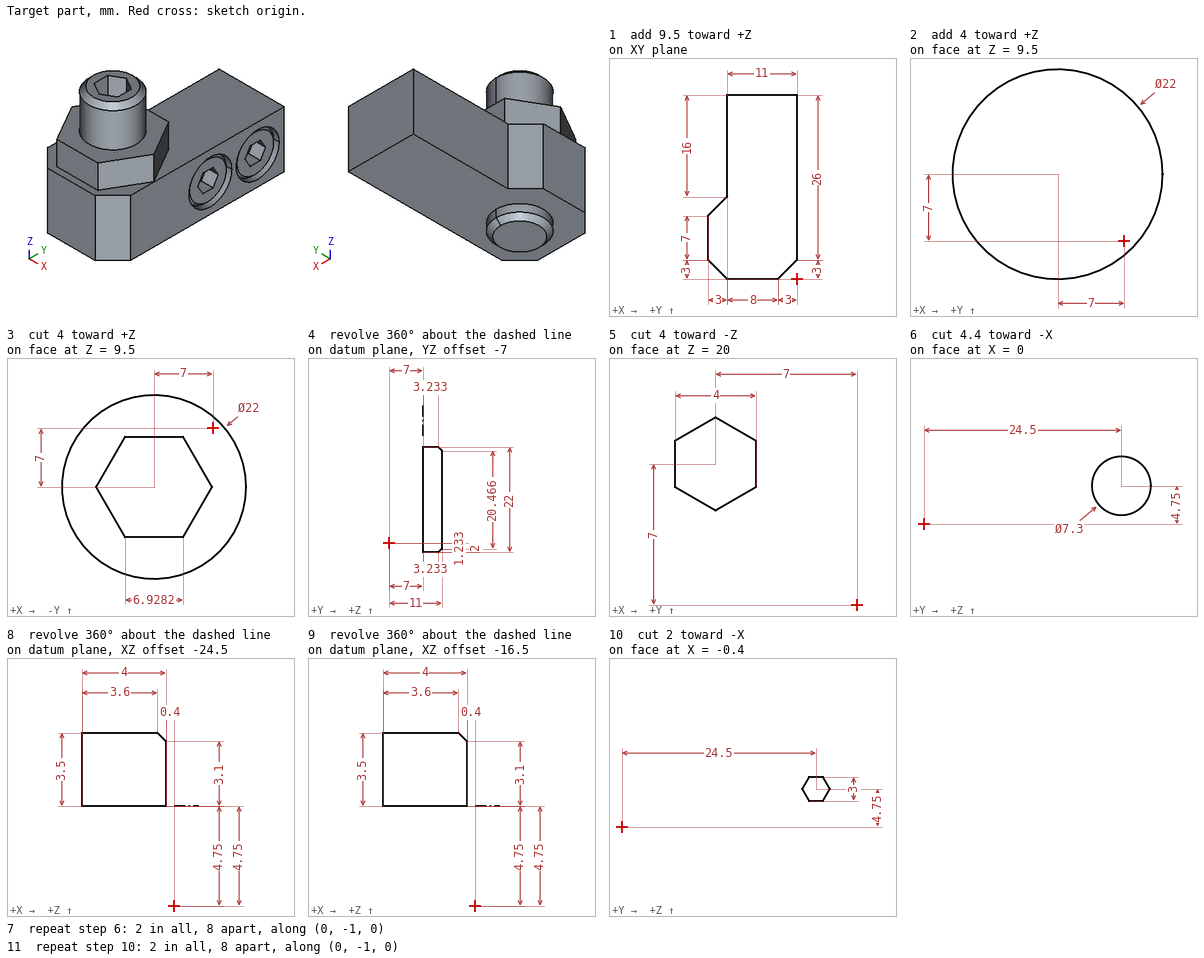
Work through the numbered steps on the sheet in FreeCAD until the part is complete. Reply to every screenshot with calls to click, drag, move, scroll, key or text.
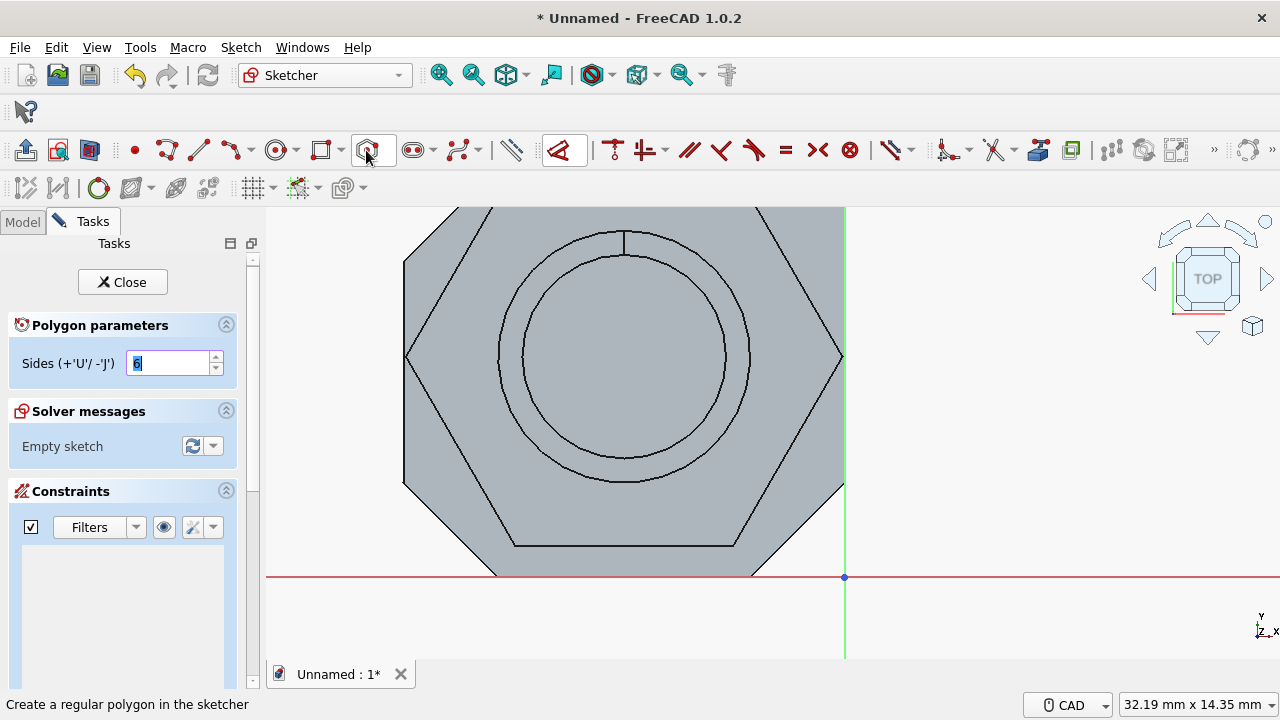
click(624, 357)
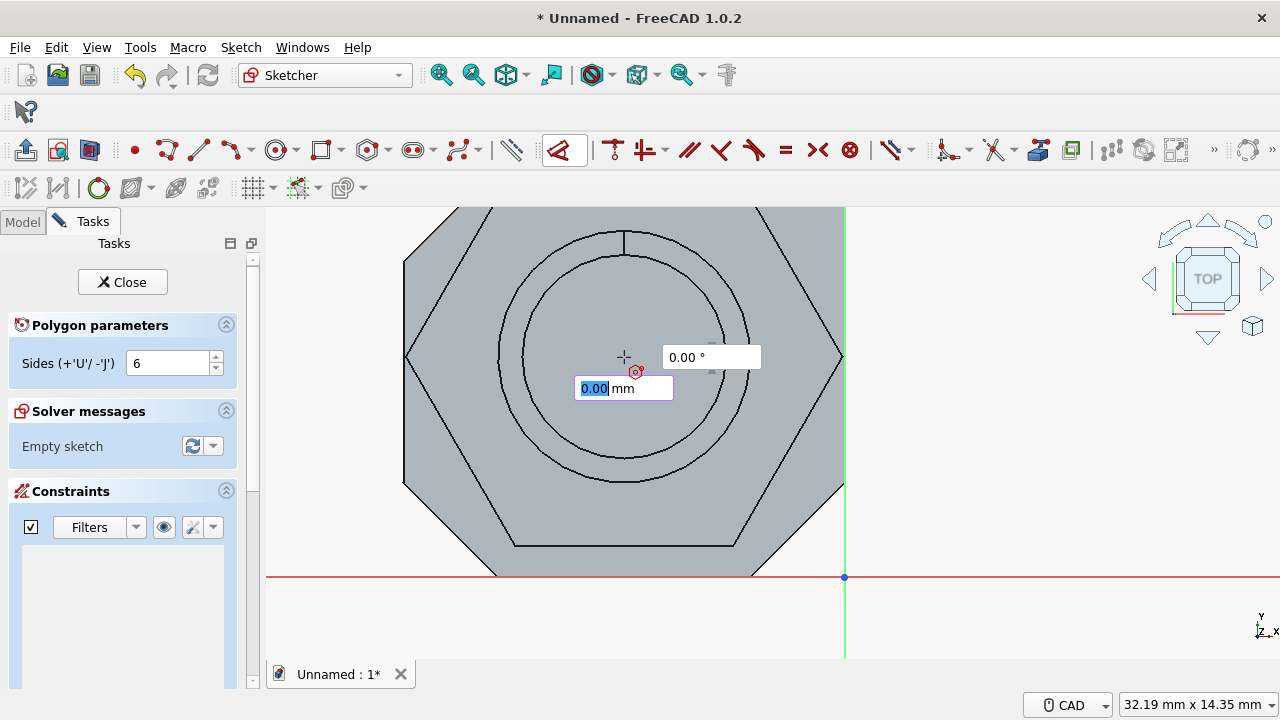
click(624, 284)
right_click(624, 284)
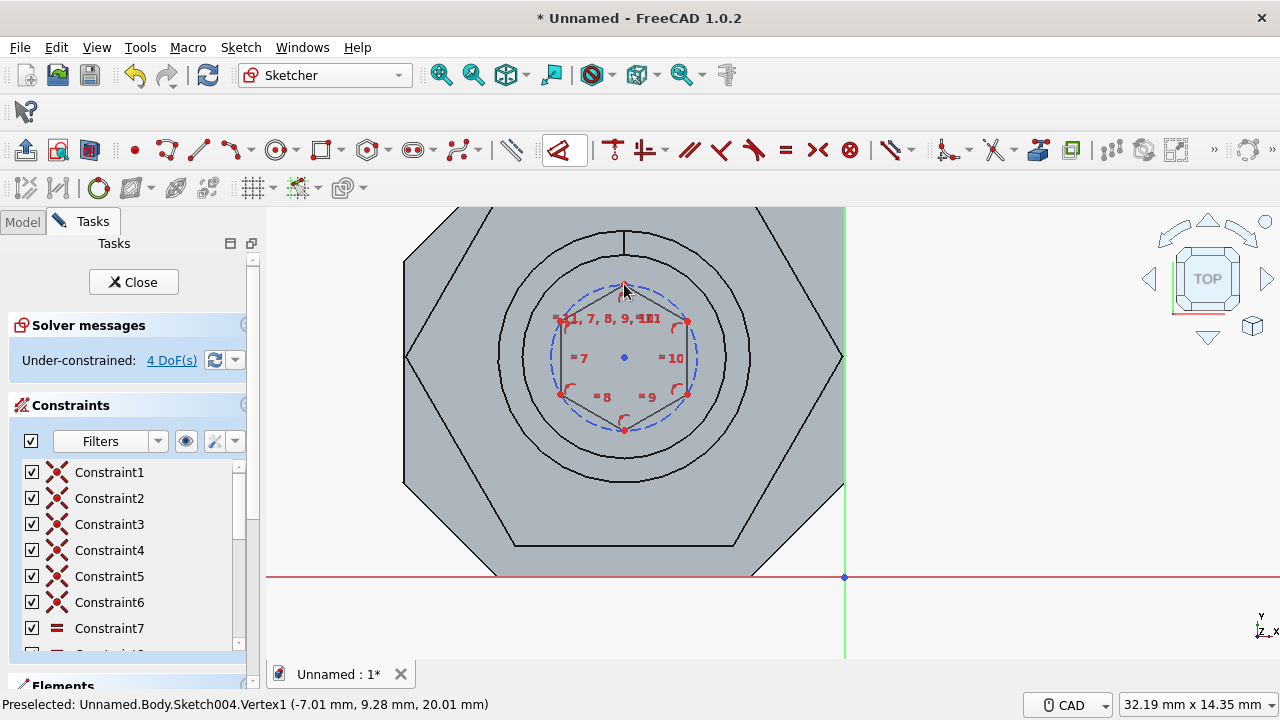
scroll(561, 351, up, 2)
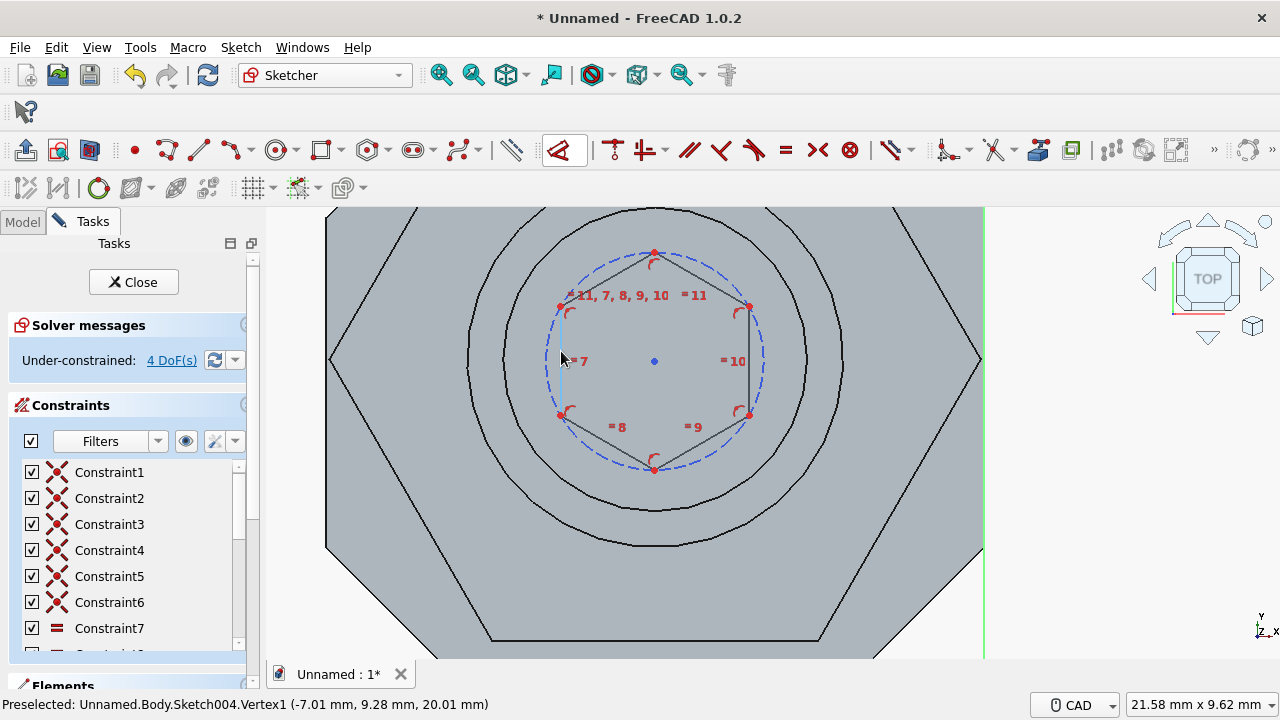
click(561, 350)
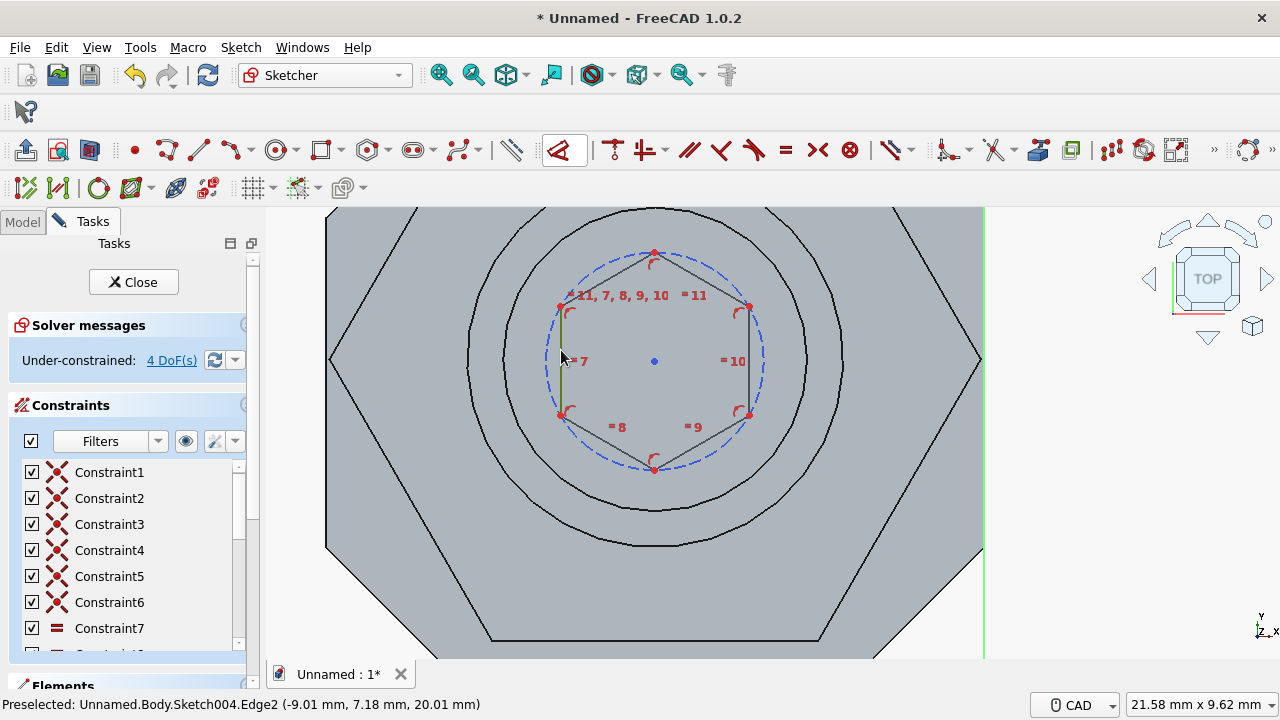
click(668, 150)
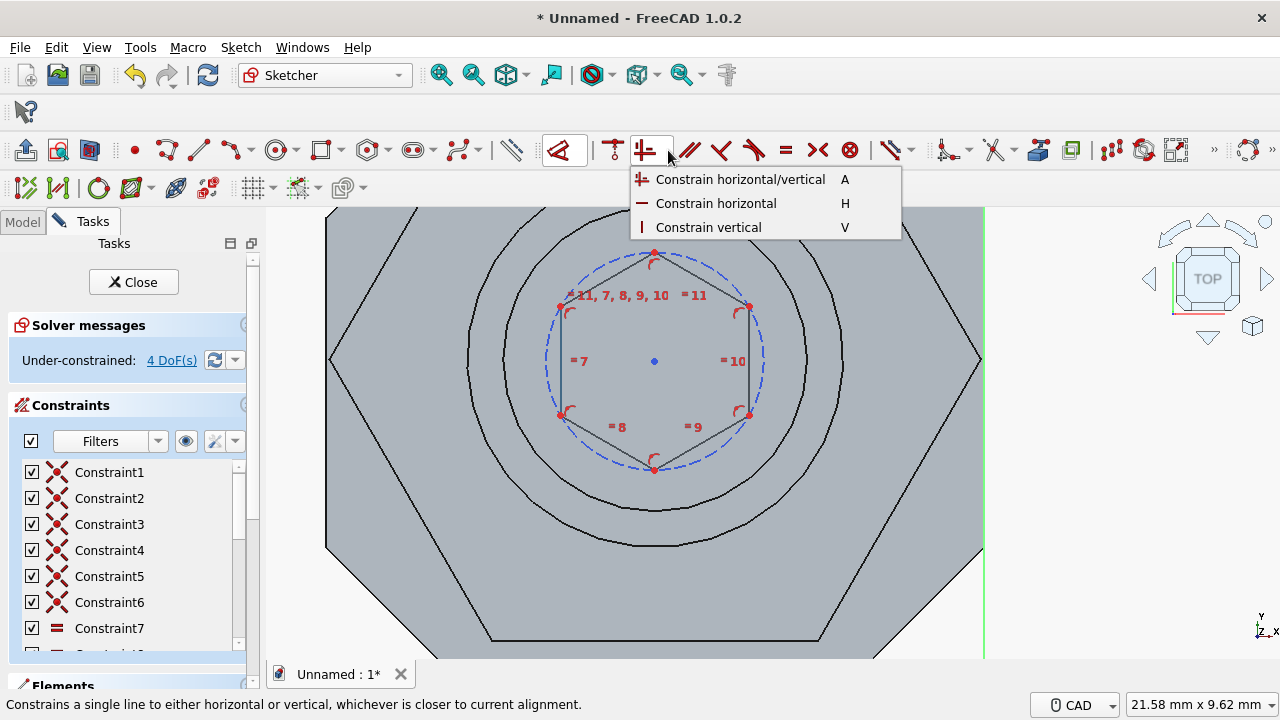
click(766, 227)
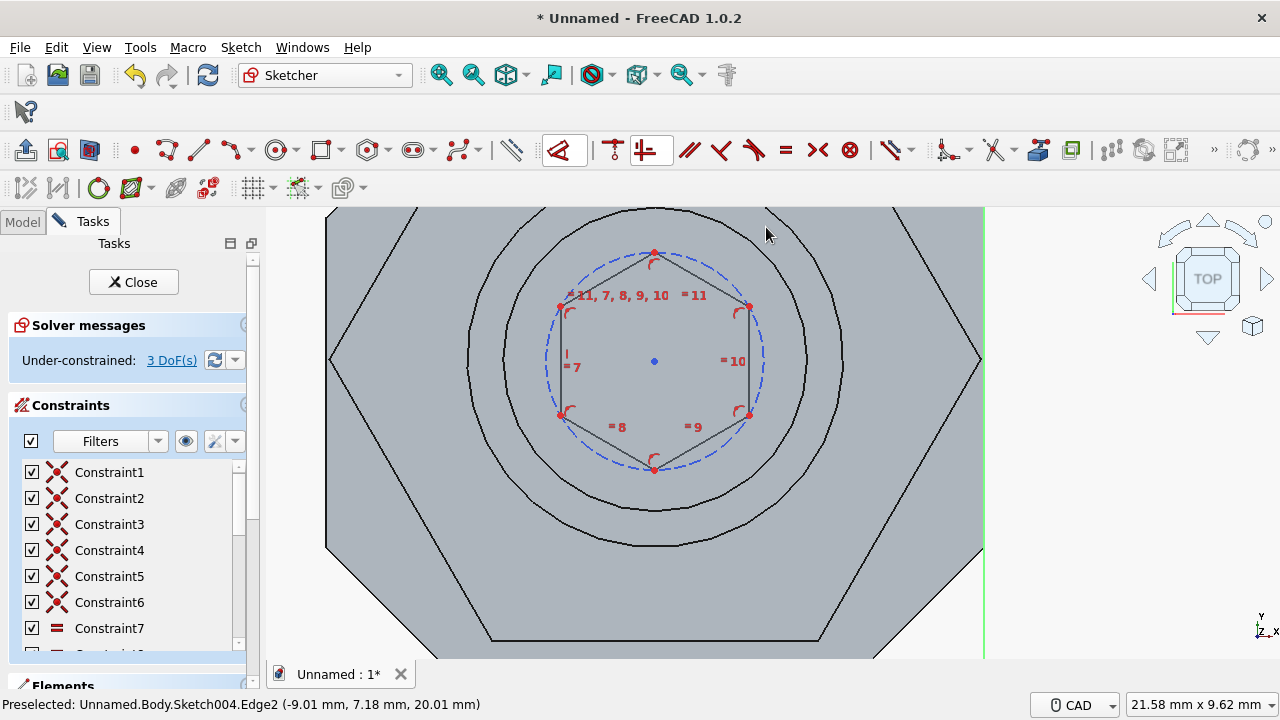
click(561, 307)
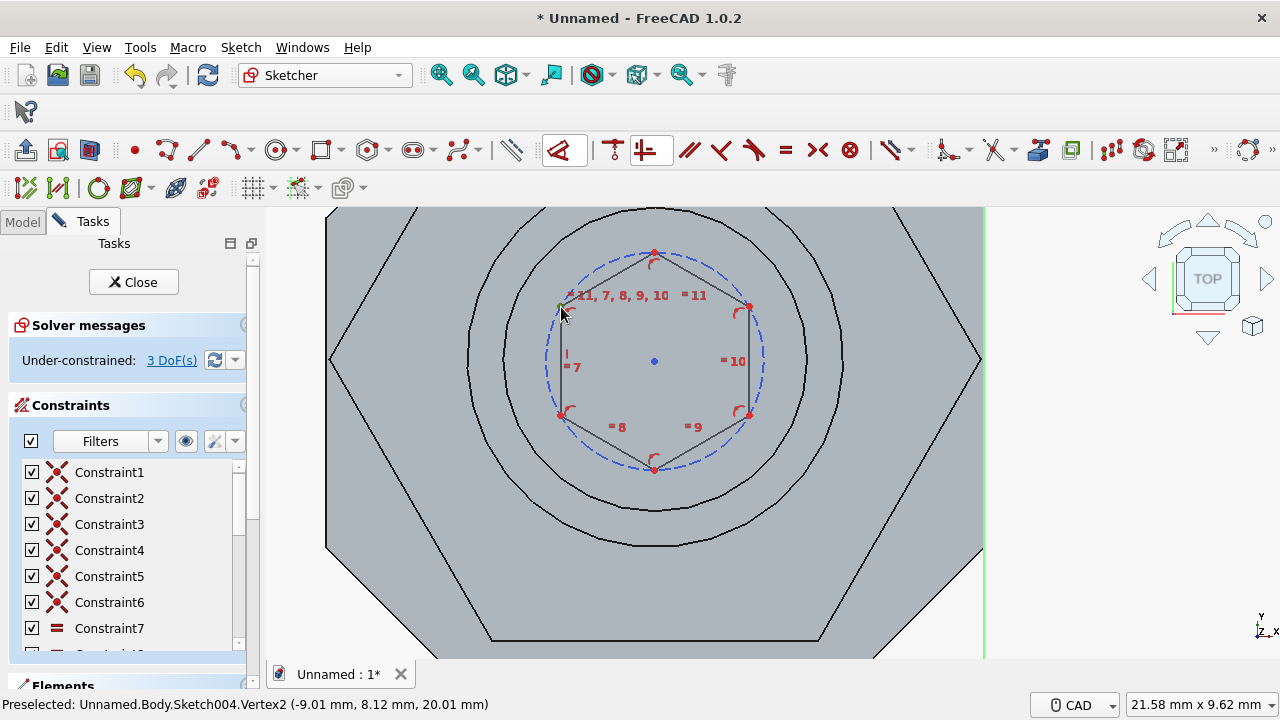
click(749, 416)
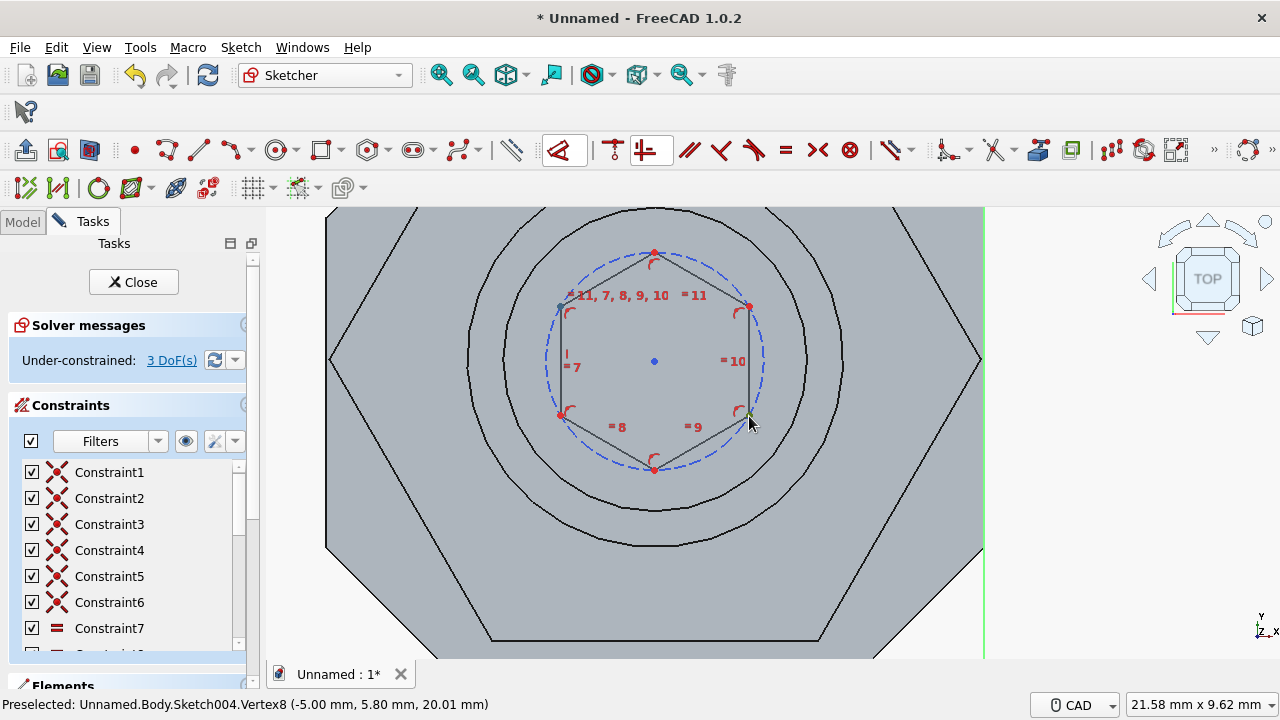
key(l)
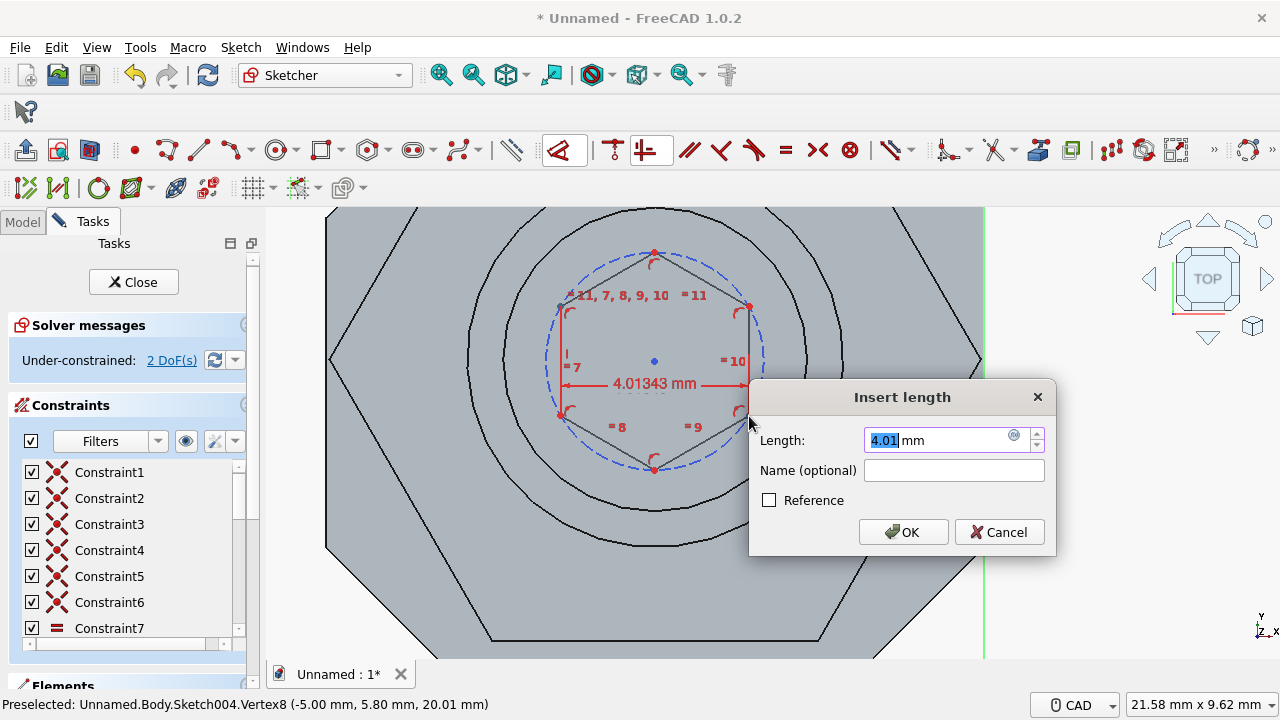
text(4)
key(Return)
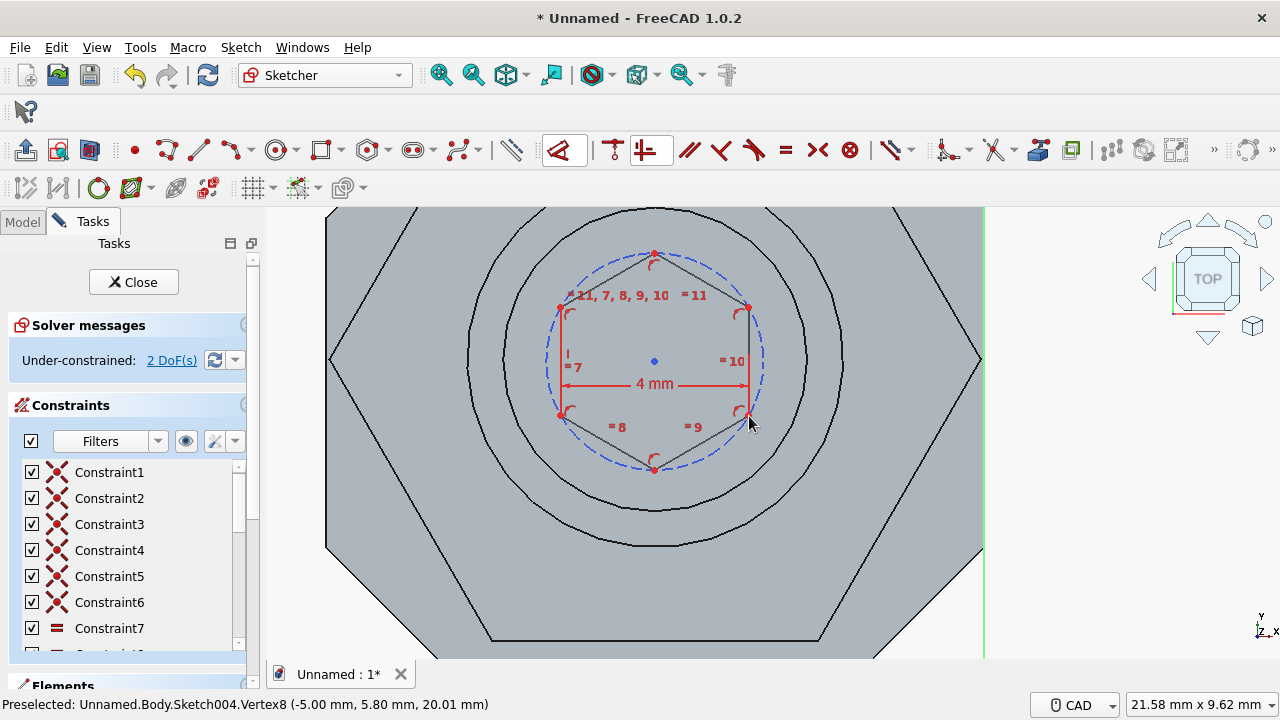
click(655, 362)